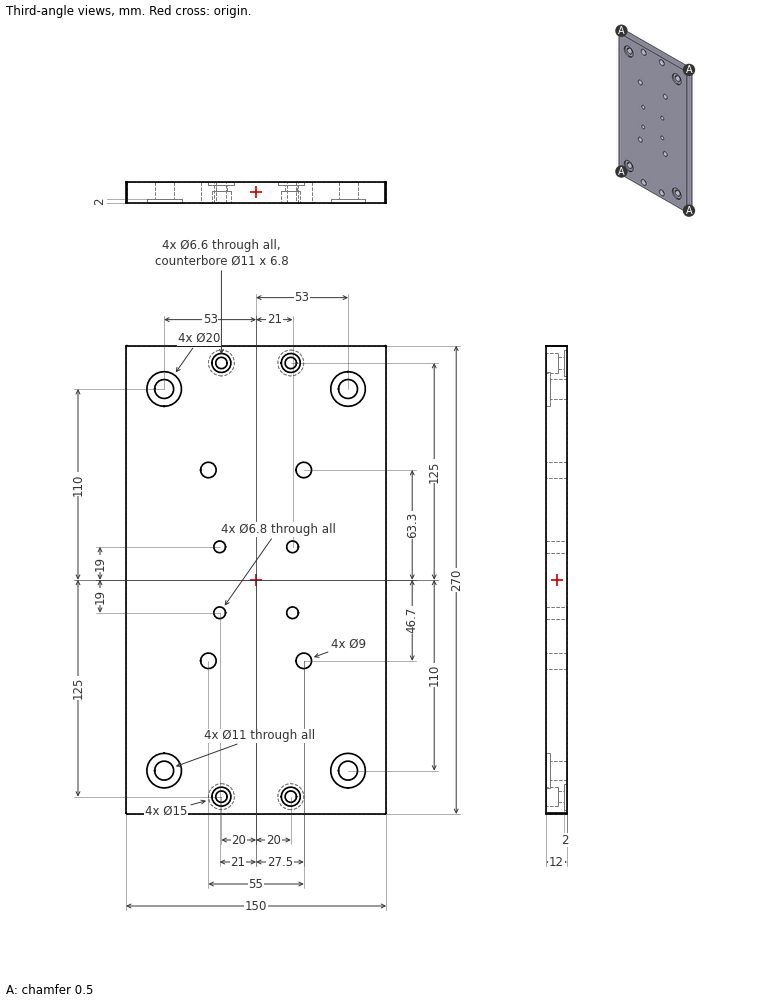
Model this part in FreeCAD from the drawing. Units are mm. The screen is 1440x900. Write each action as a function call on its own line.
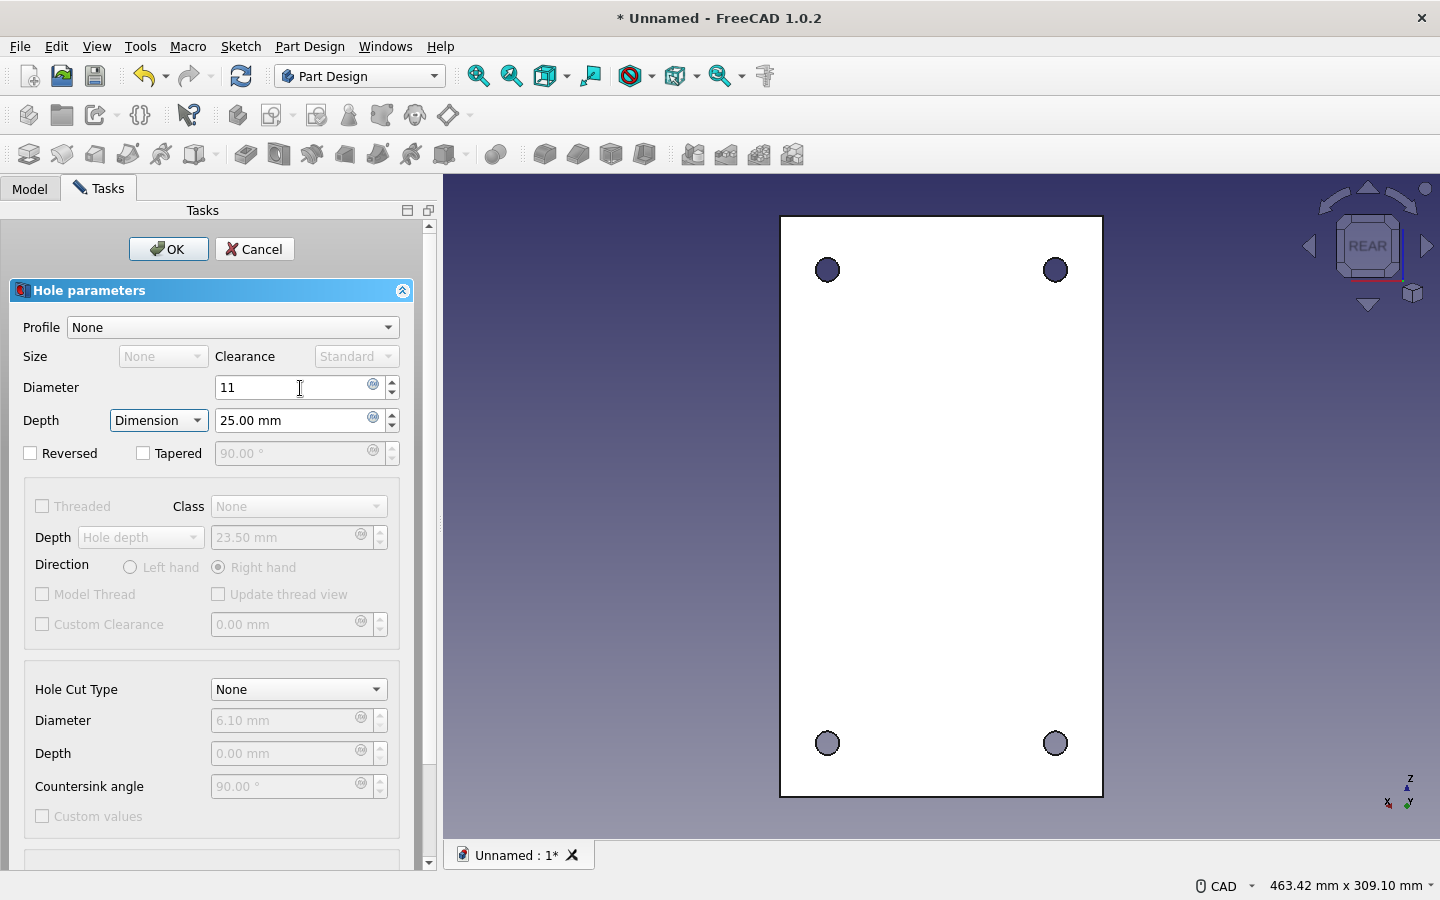
click(160, 420)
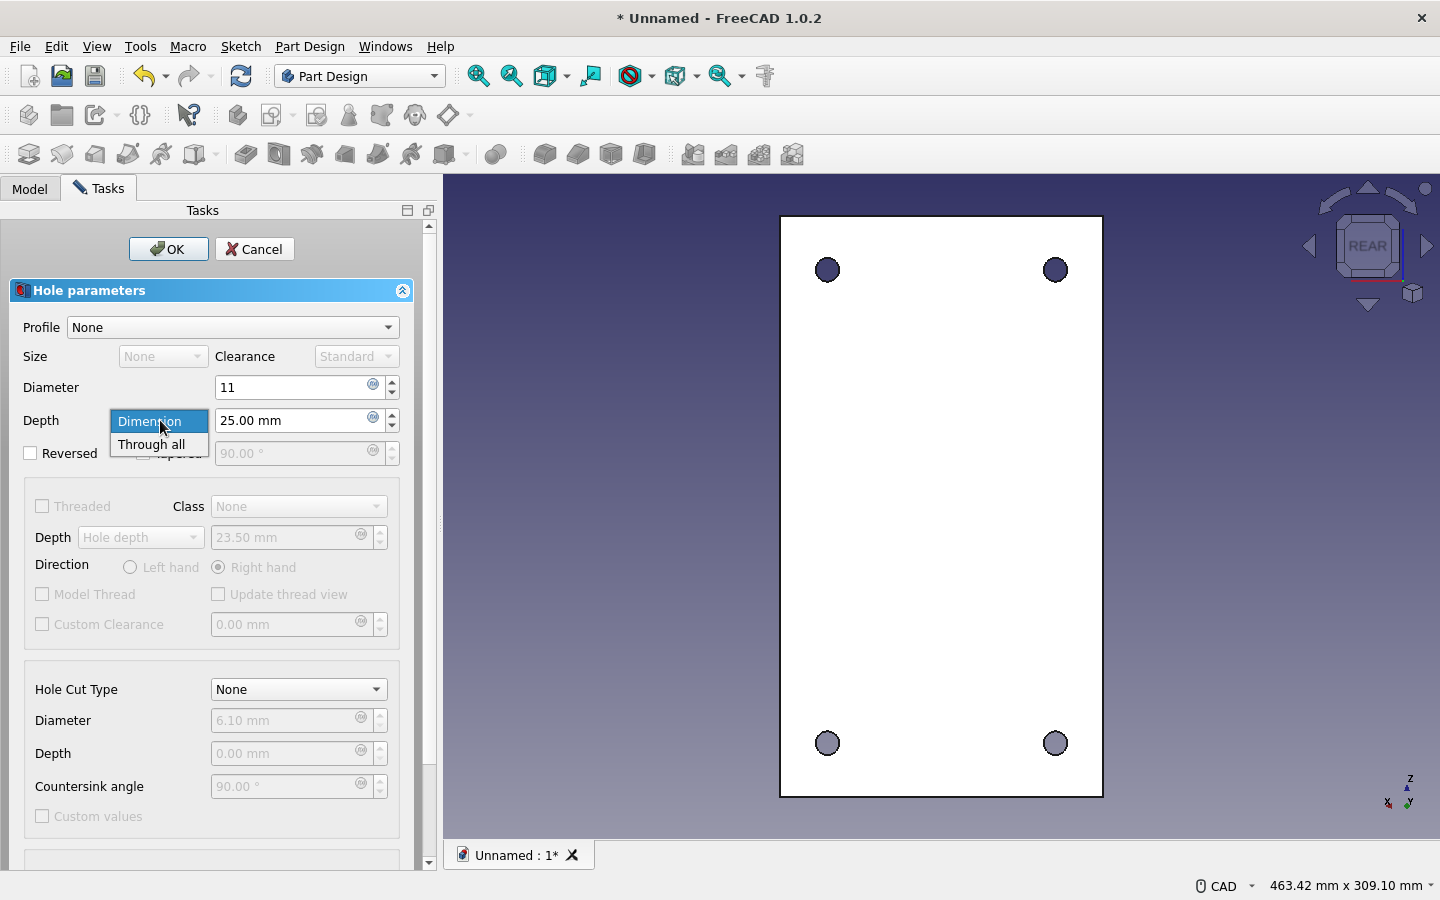
click(158, 444)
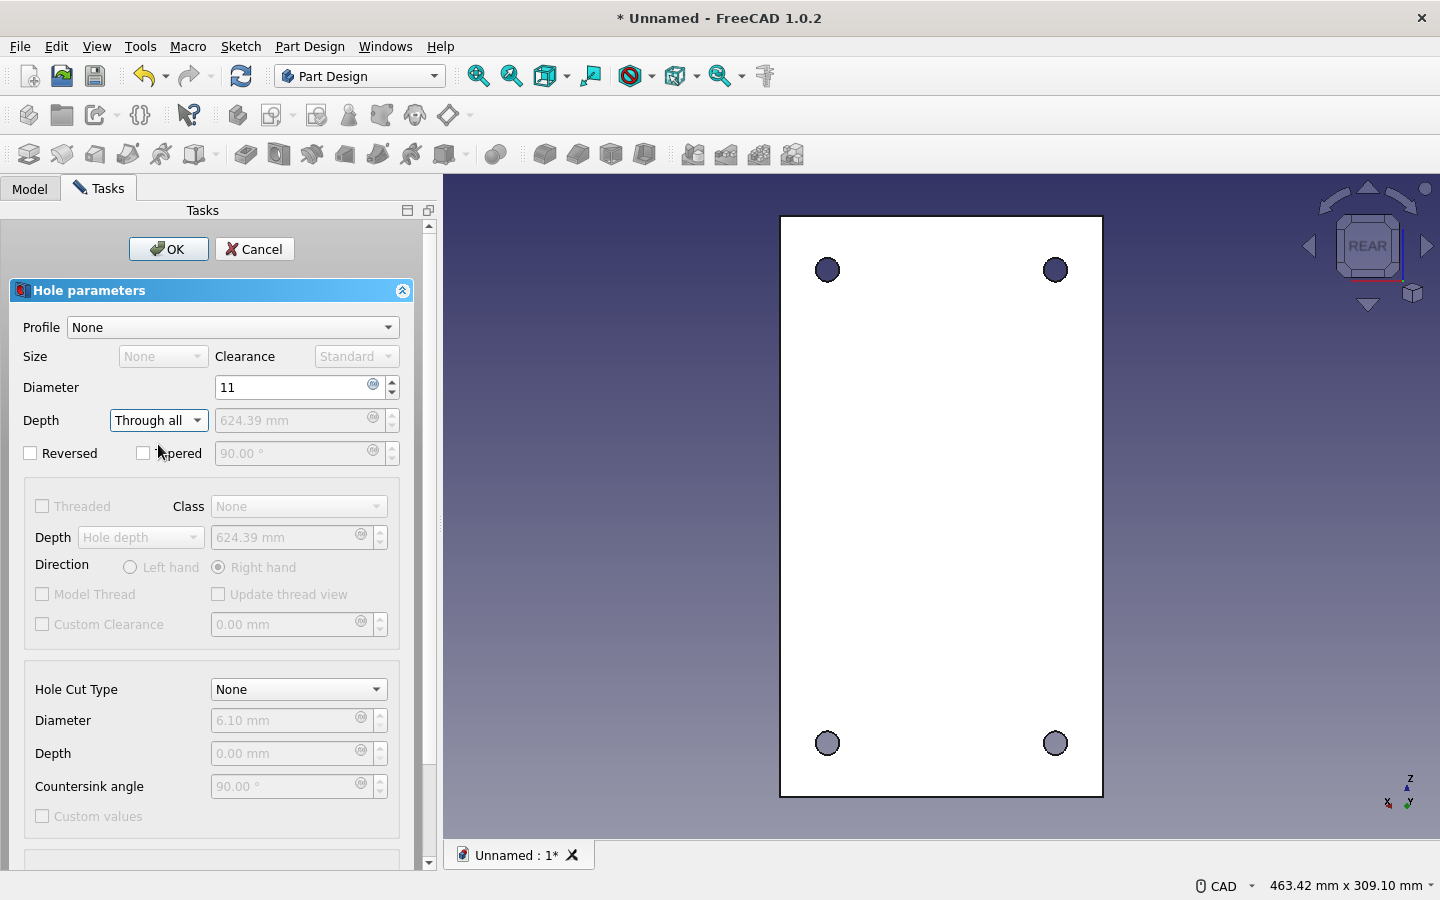
click(169, 249)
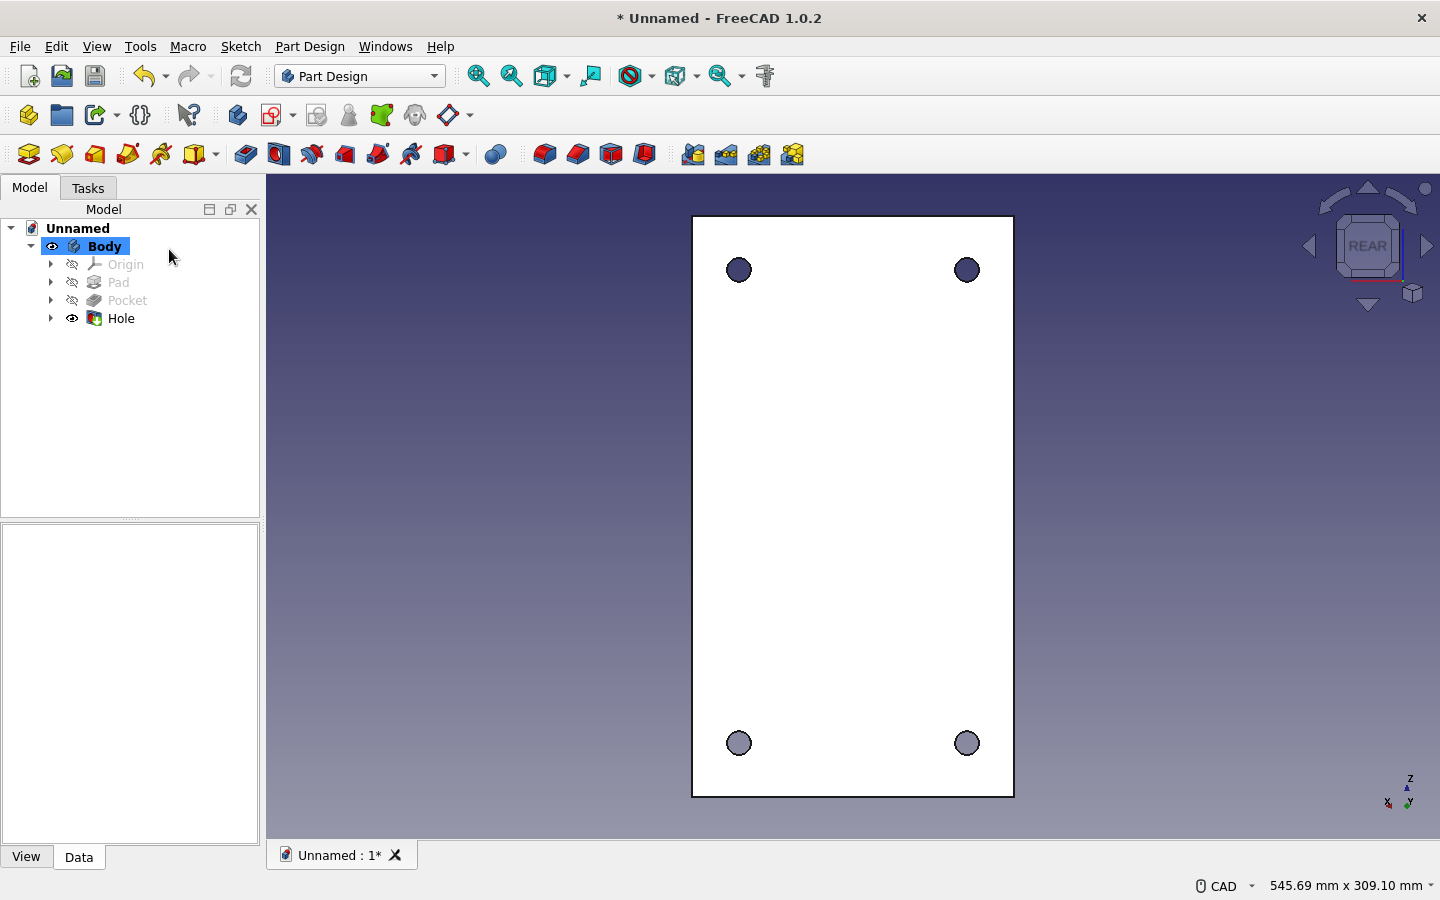
click(853, 423)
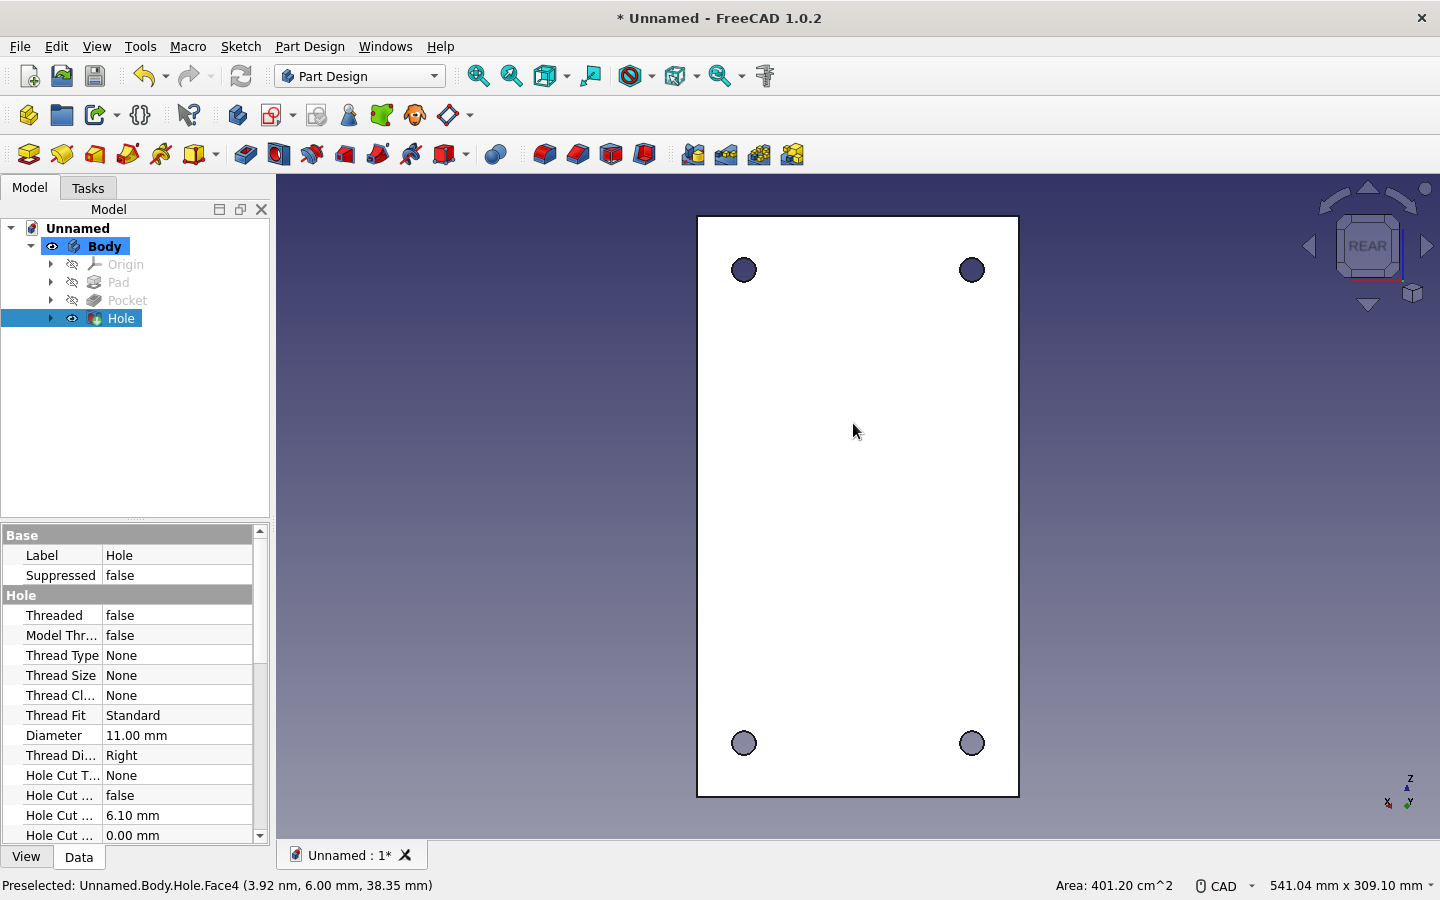
click(270, 116)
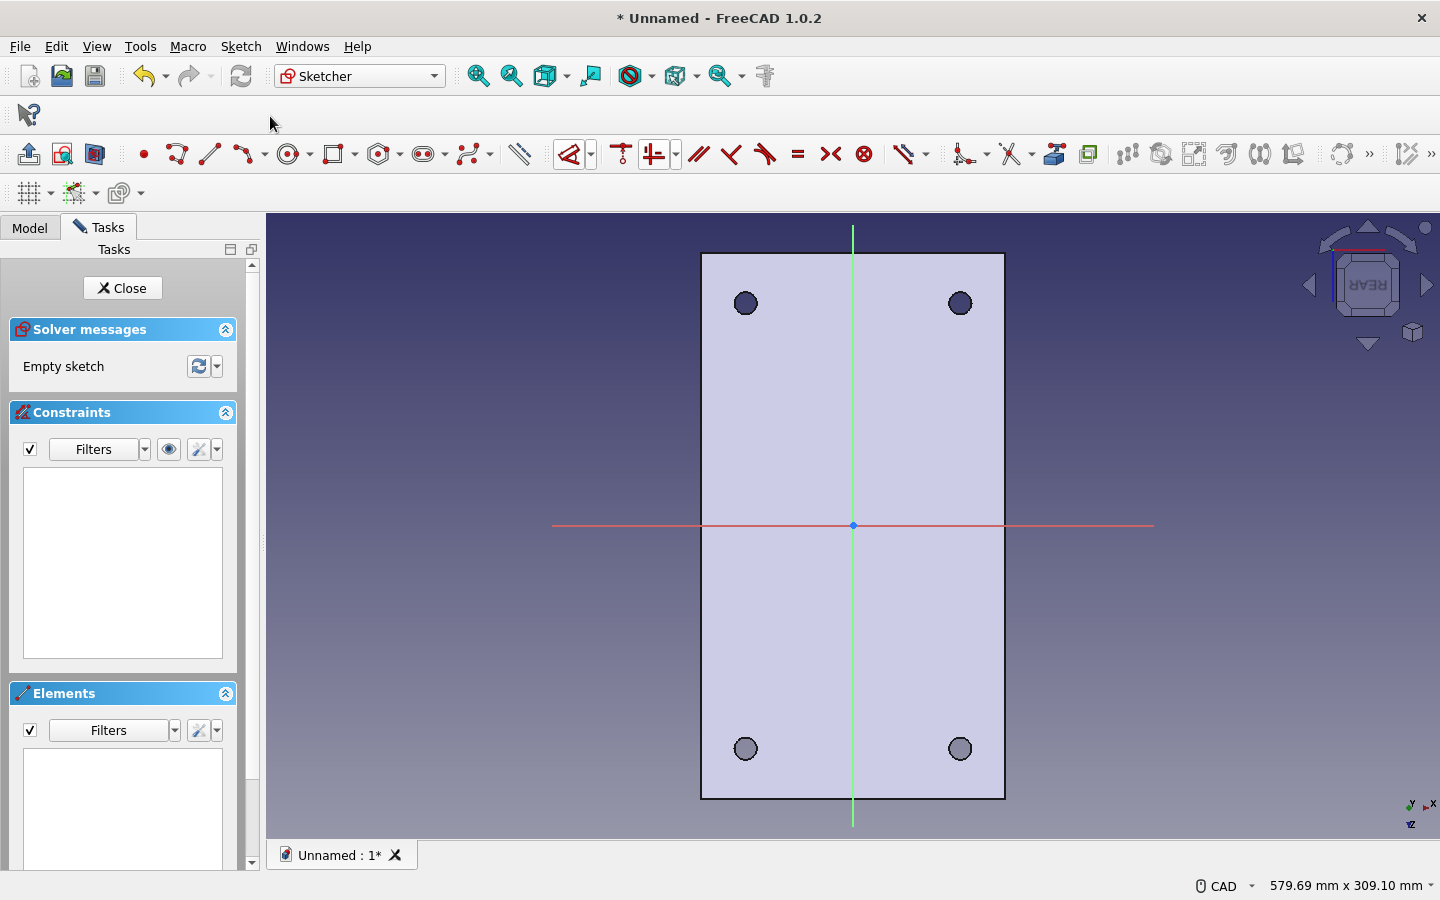
scroll(475, 526, down, 1)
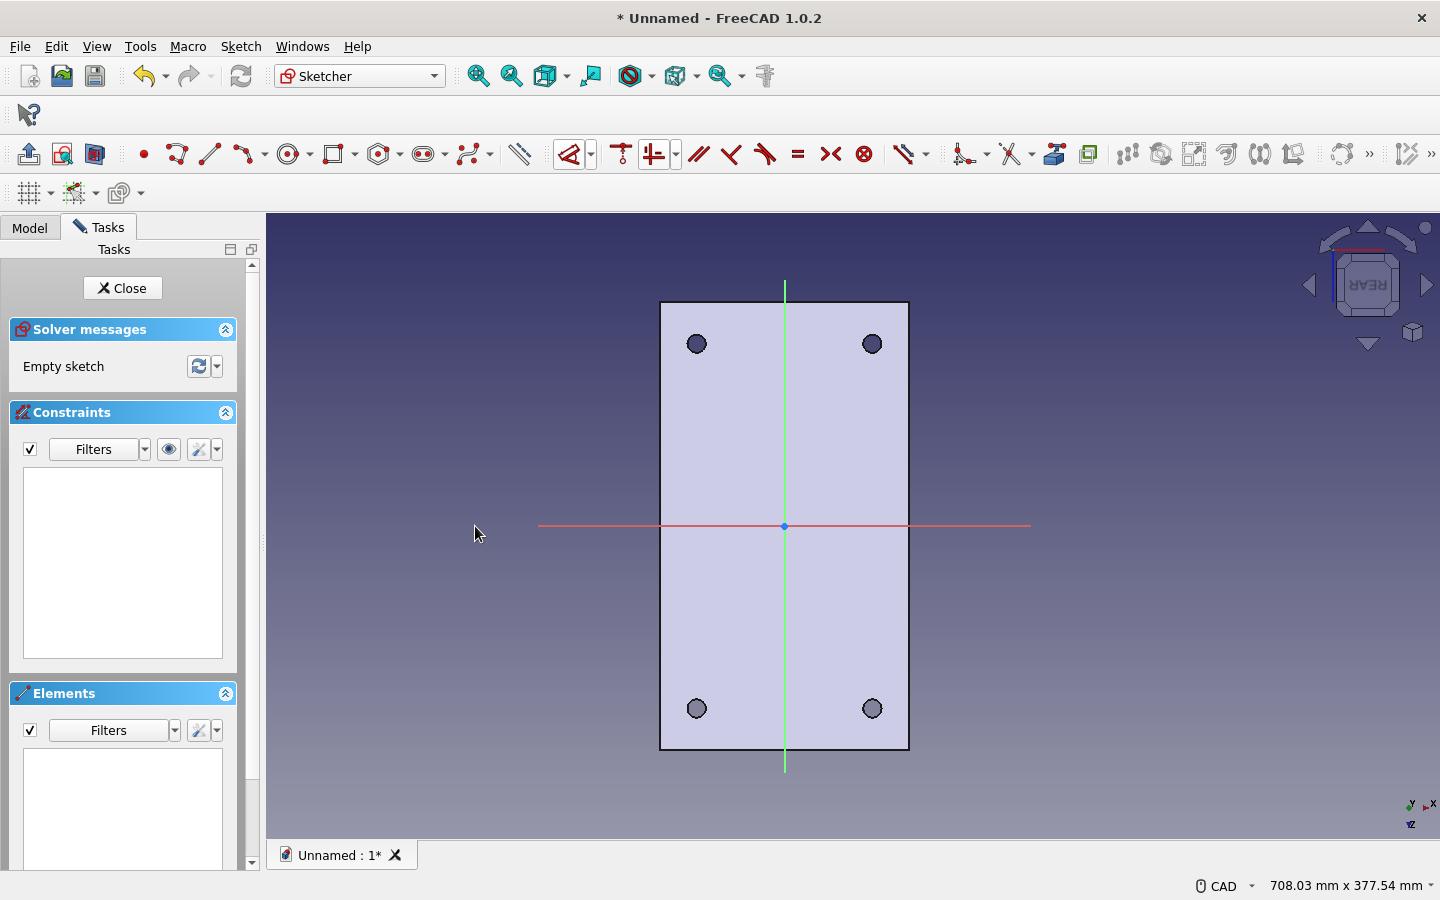
key(g)
key(c)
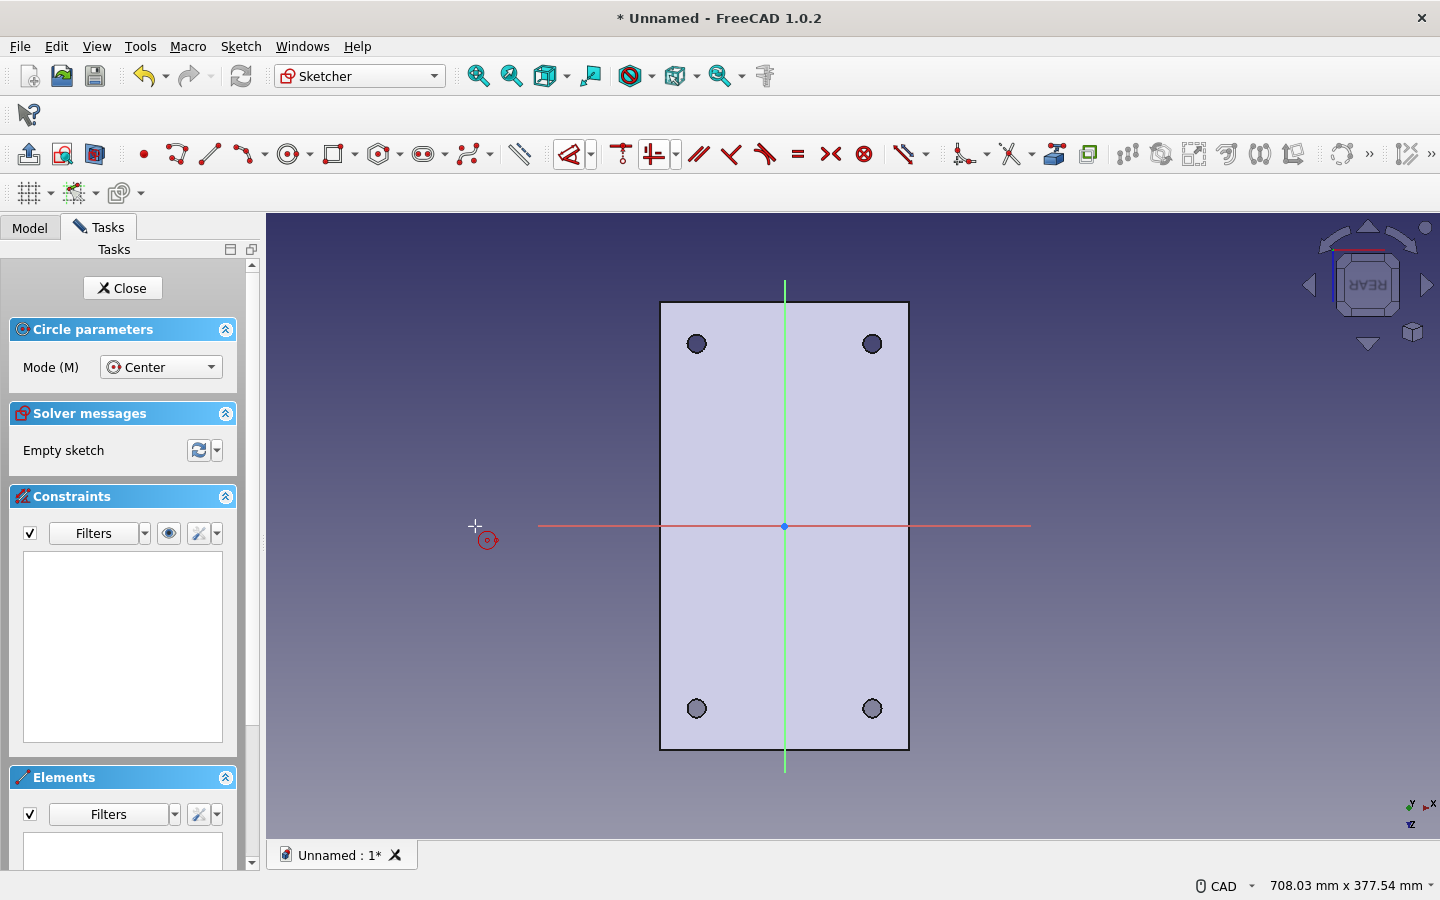
scroll(751, 319, up, 4)